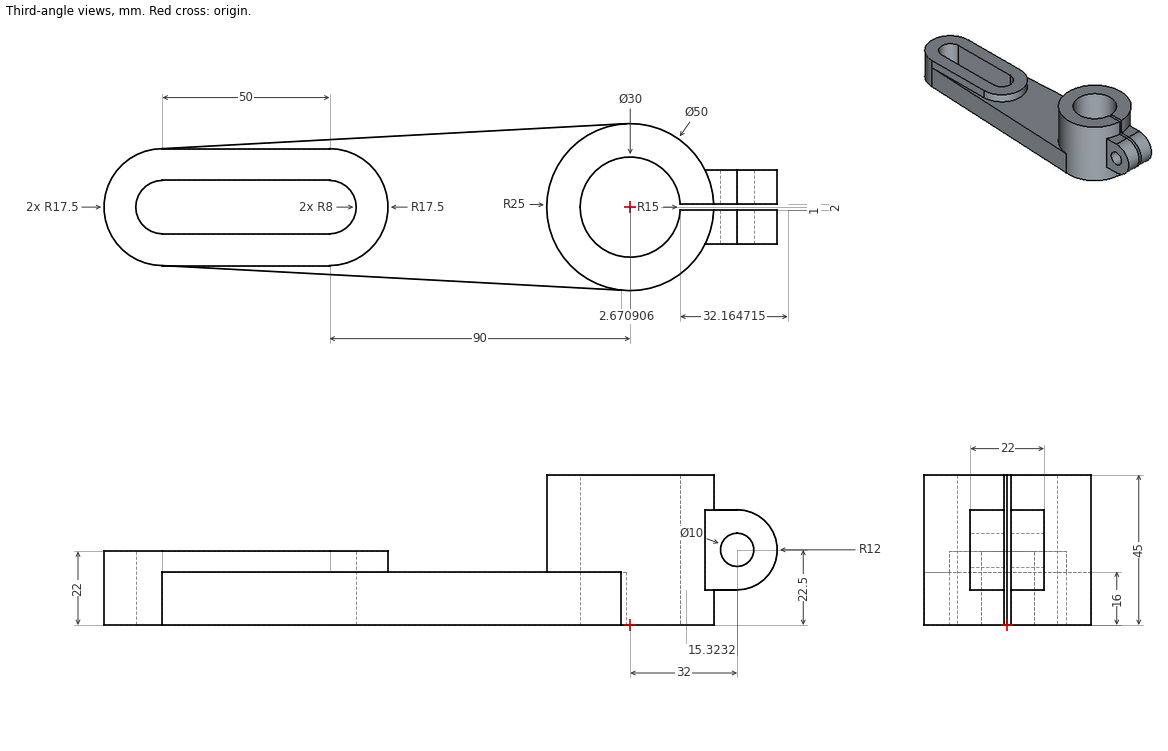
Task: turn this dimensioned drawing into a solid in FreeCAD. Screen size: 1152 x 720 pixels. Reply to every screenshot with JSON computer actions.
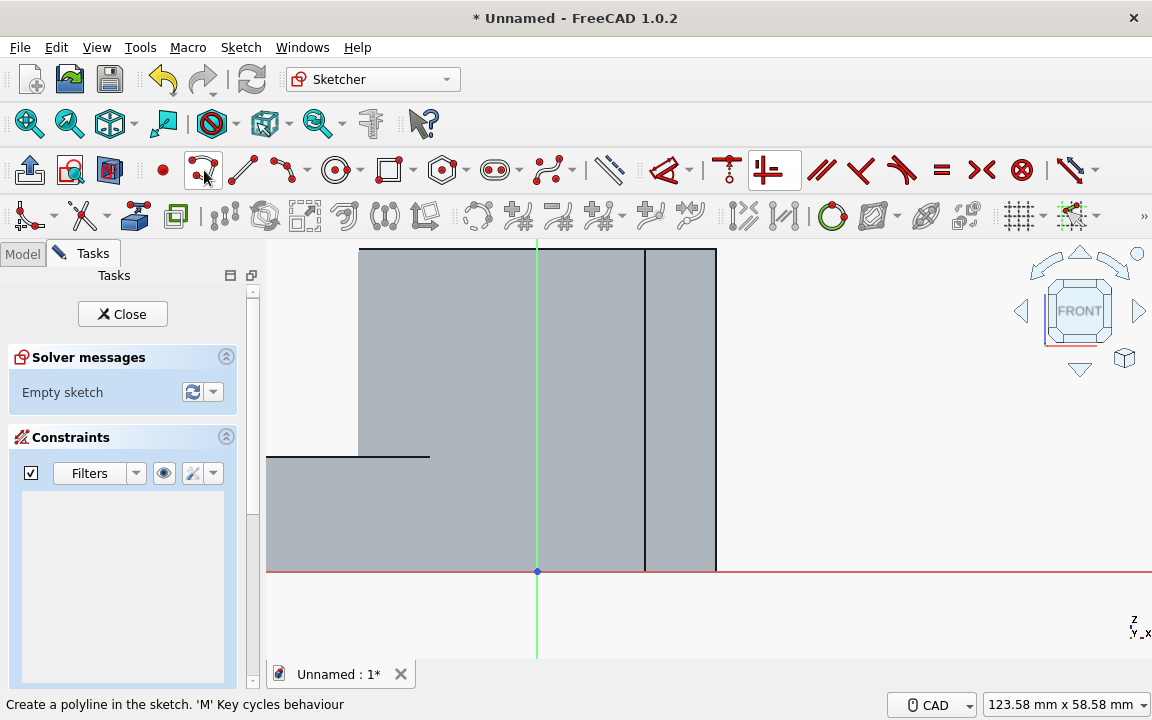
{"action": "left_click", "coordinate": [767, 497]}
{"action": "left_click", "coordinate": [657, 497]}
{"action": "left_click", "coordinate": [657, 325]}
{"action": "left_click", "coordinate": [767, 325]}
{"action": "right_click", "coordinate": [767, 325]}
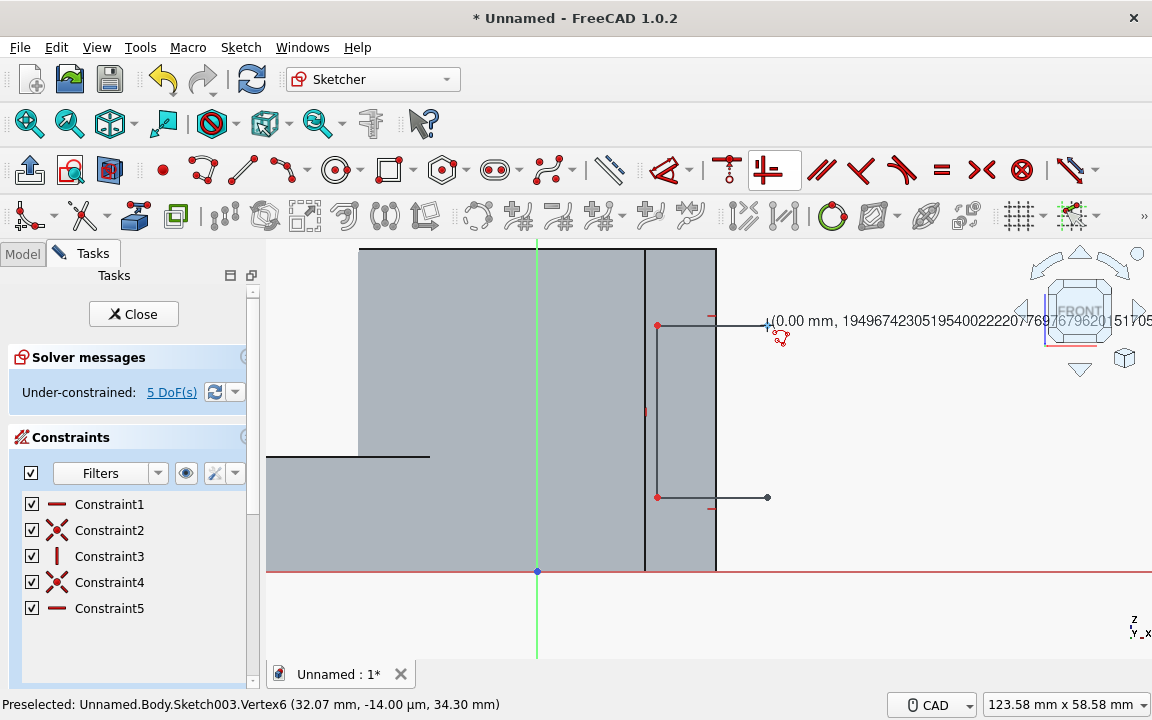
{"action": "left_click", "coordinate": [284, 170]}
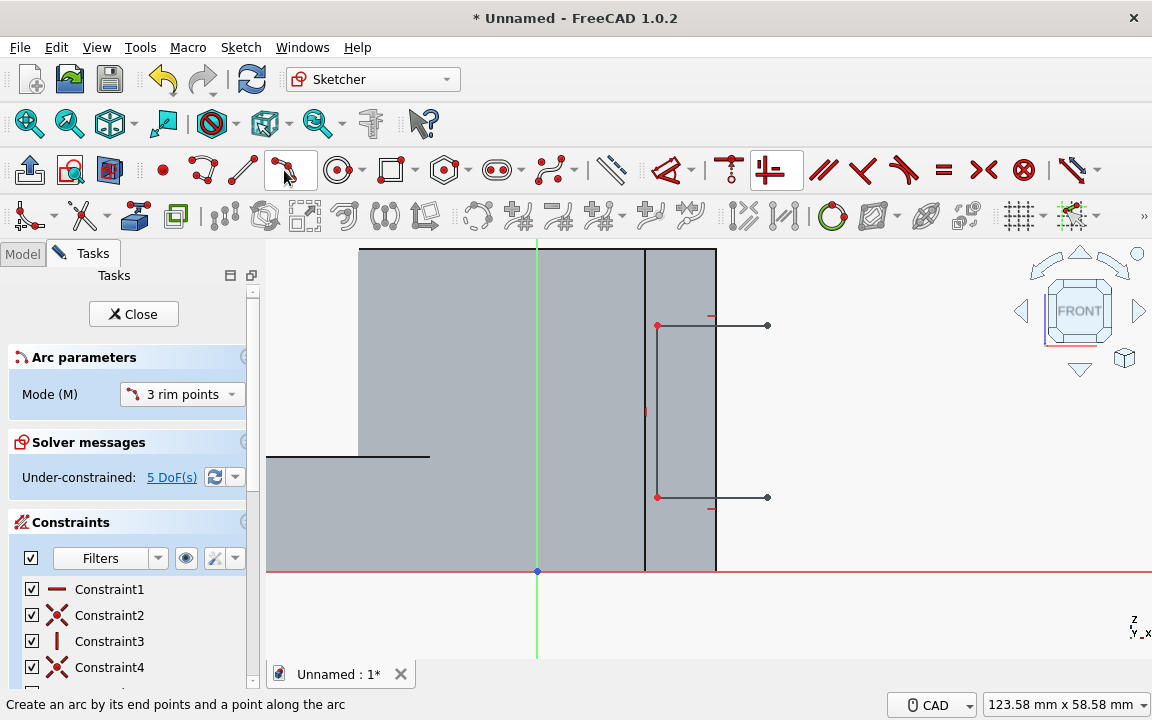
{"action": "left_click", "coordinate": [767, 326]}
{"action": "left_click", "coordinate": [767, 498]}
{"action": "left_click", "coordinate": [853, 411]}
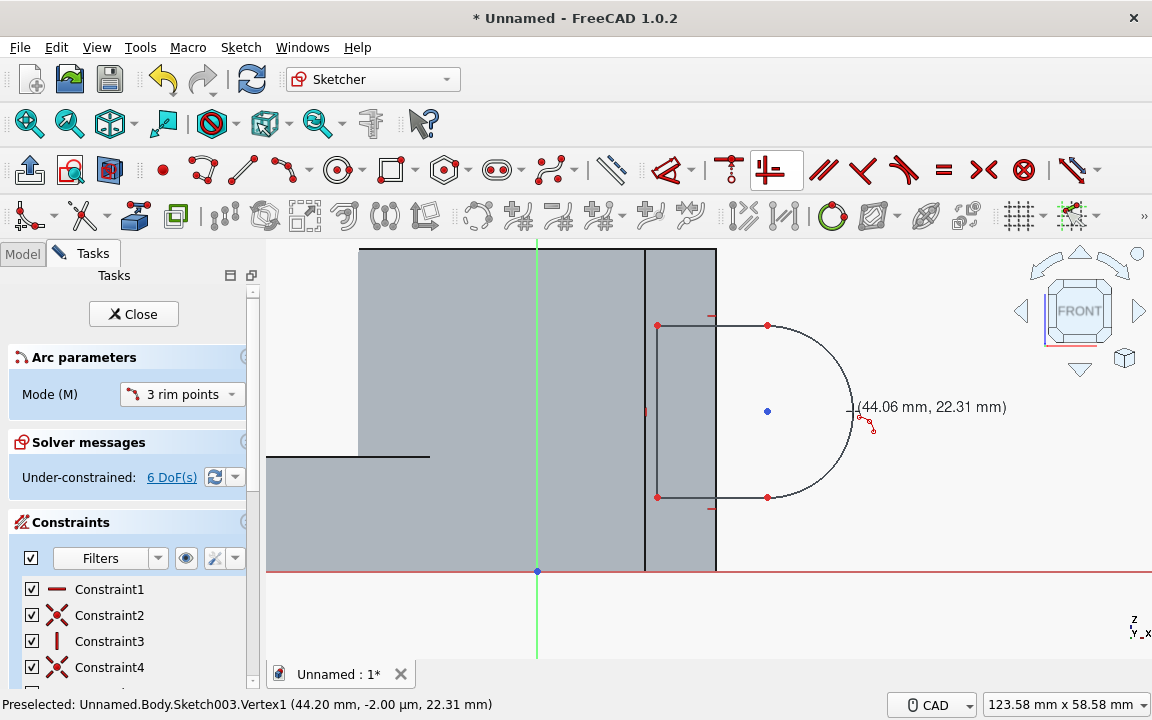
{"action": "left_click", "coordinate": [338, 170]}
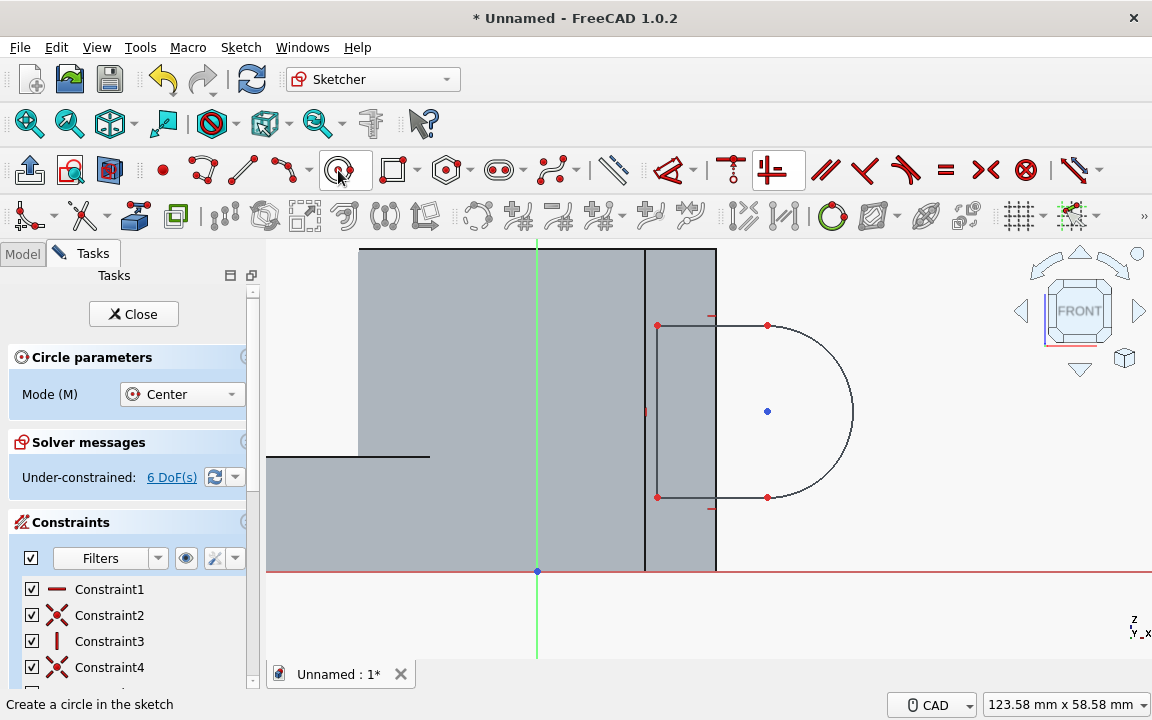
{"action": "left_click", "coordinate": [767, 411]}
{"action": "left_click", "coordinate": [792, 385]}
{"action": "key", "text": "Escape"}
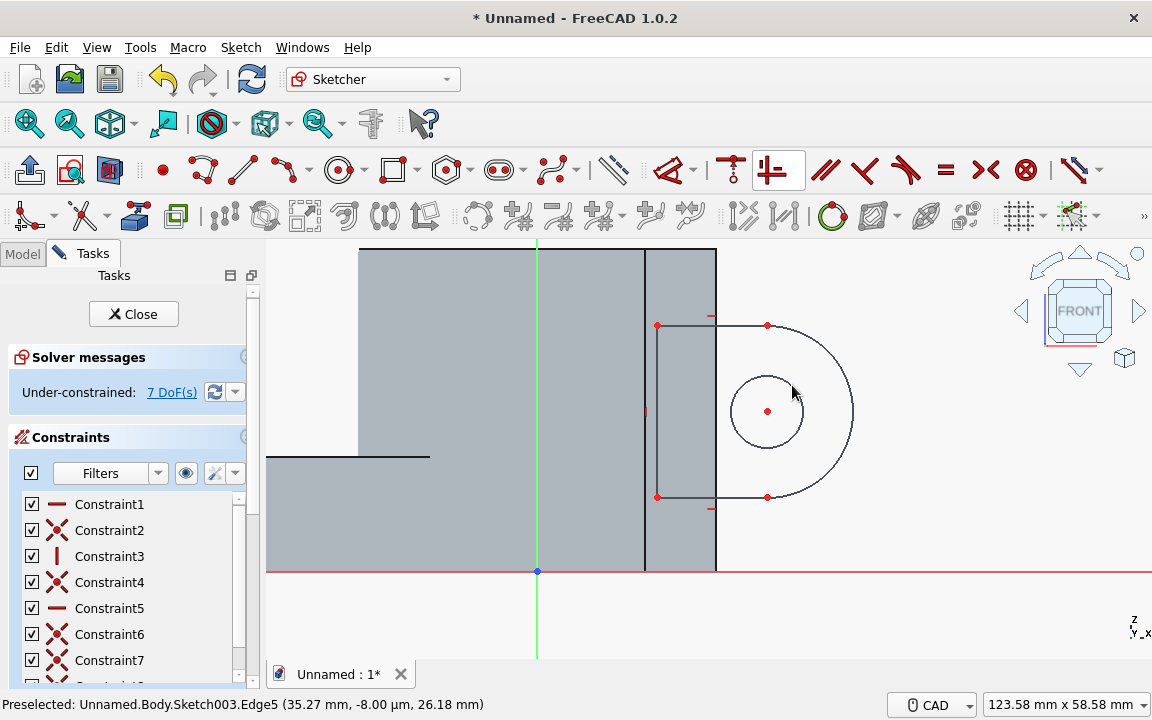
{"action": "left_click", "coordinate": [734, 498]}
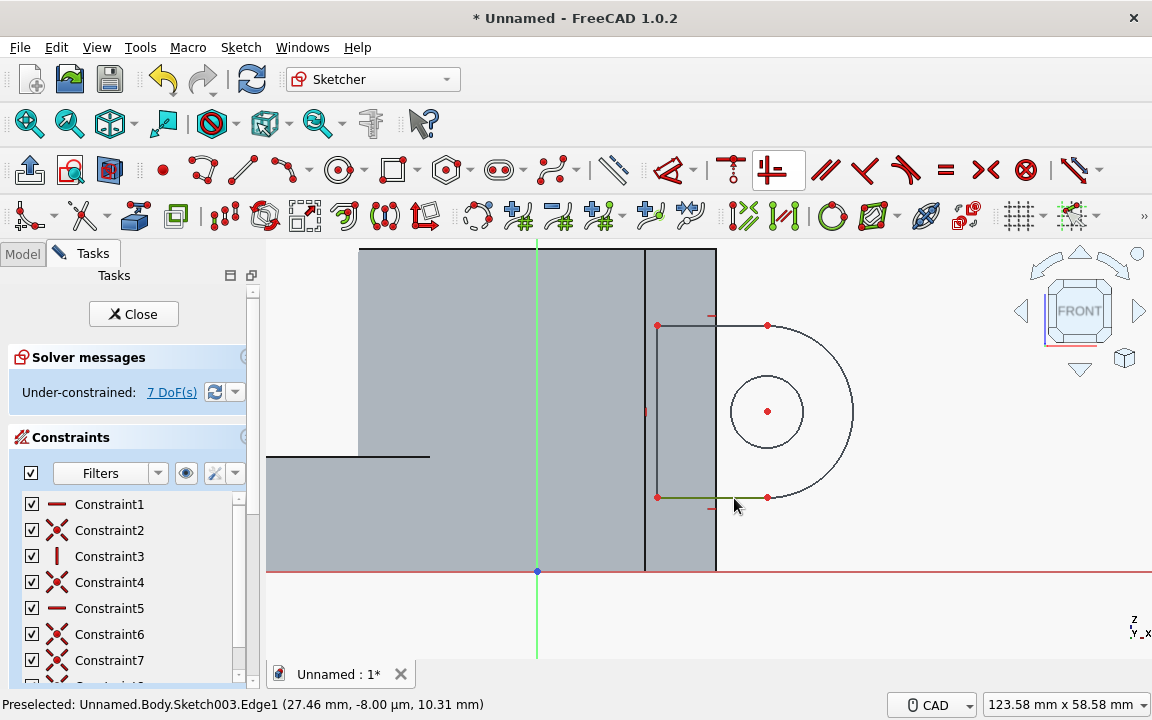
{"action": "left_click", "coordinate": [837, 463]}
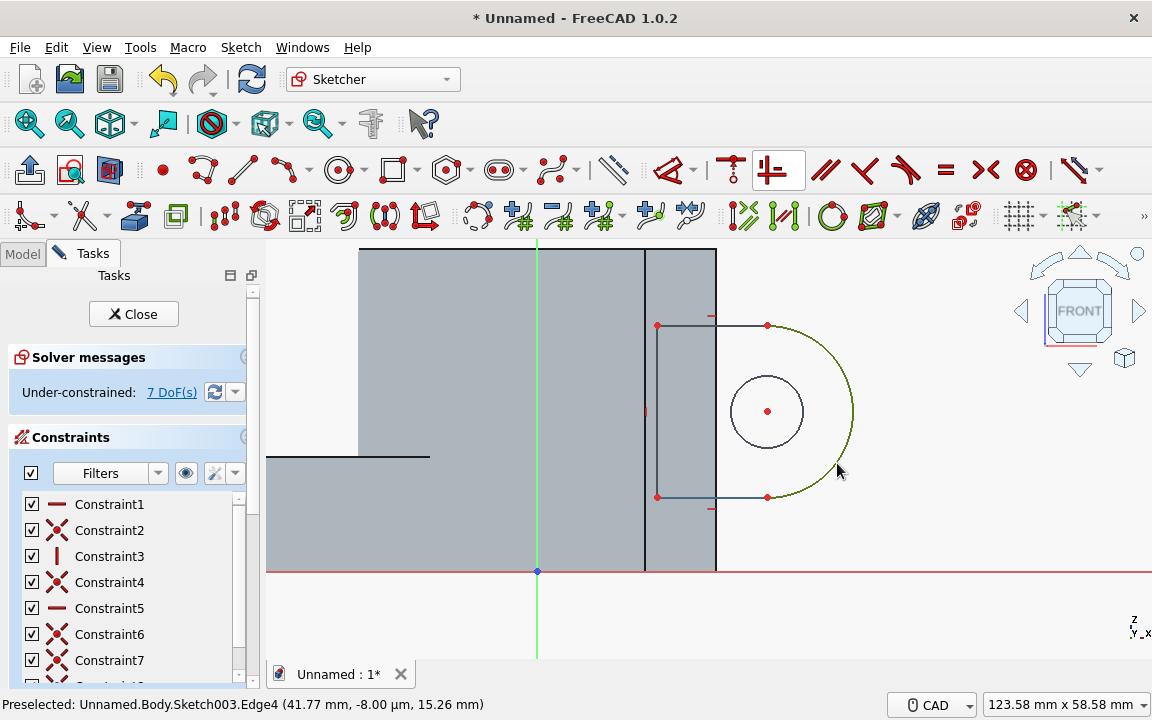
{"action": "left_click", "coordinate": [906, 170]}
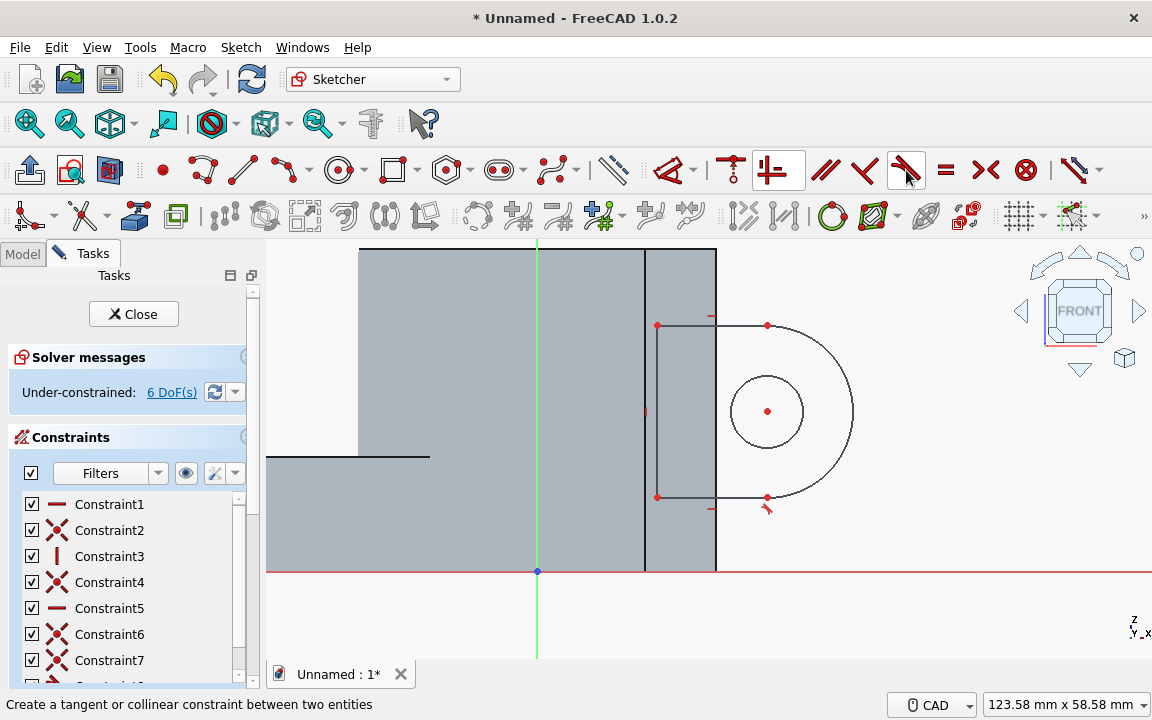
{"action": "left_click", "coordinate": [690, 326]}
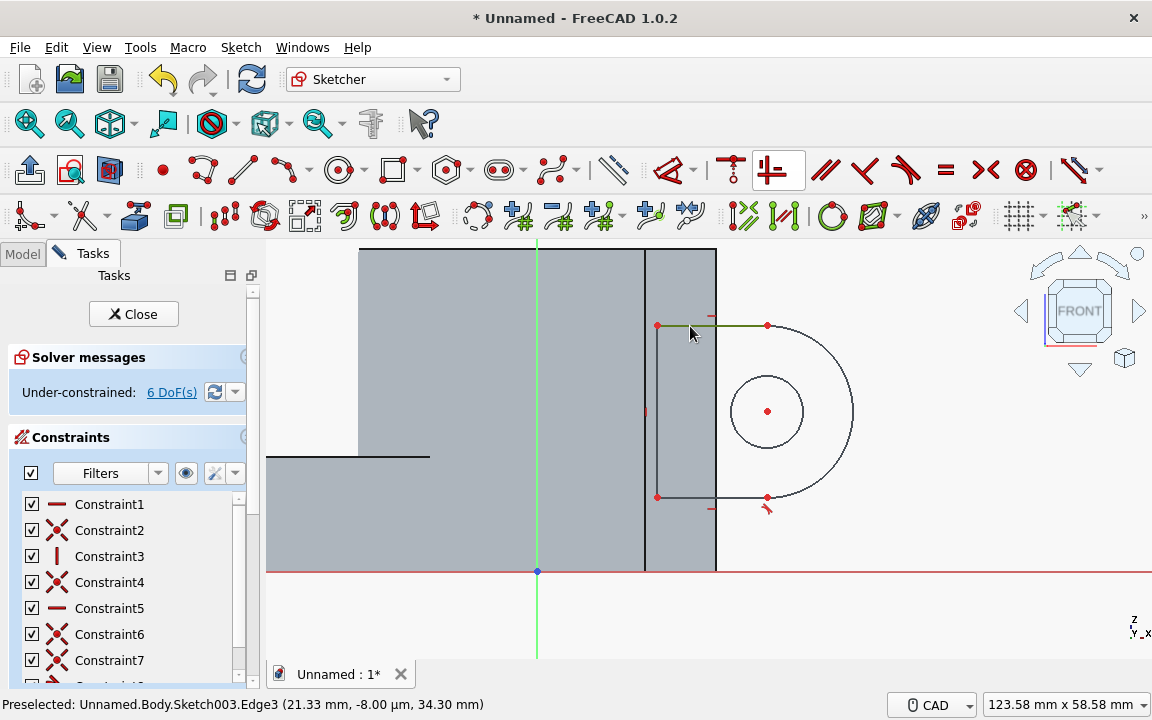
{"action": "left_click", "coordinate": [837, 463]}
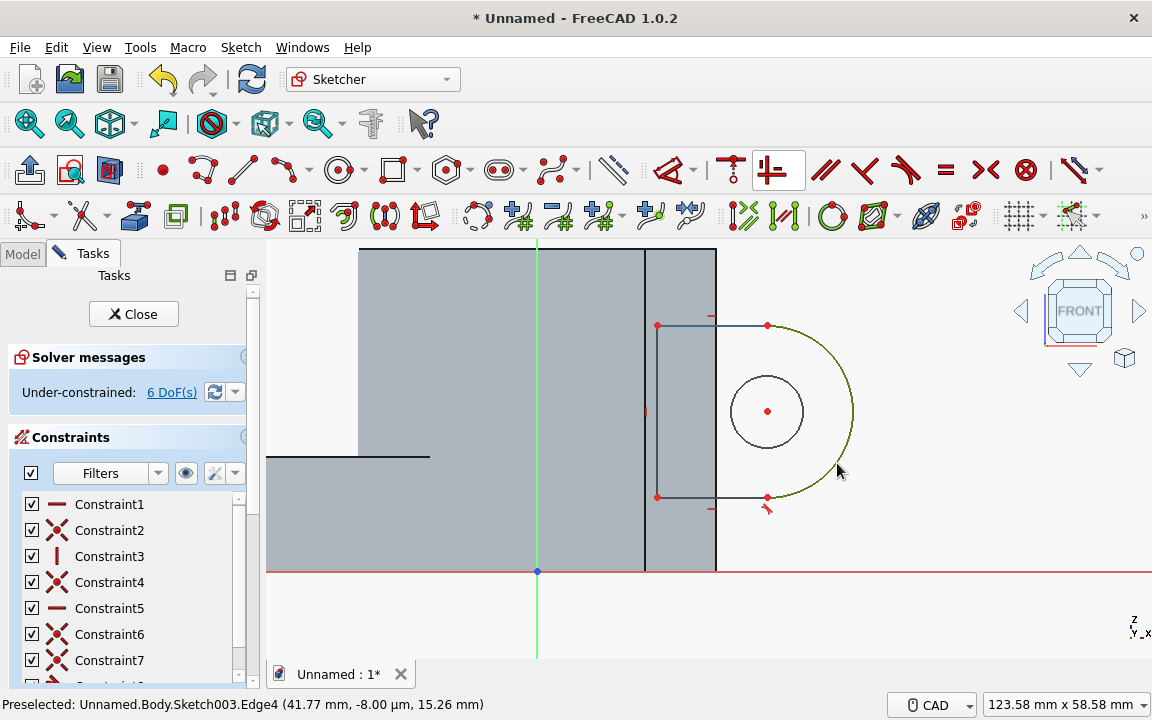
{"action": "left_click", "coordinate": [906, 170]}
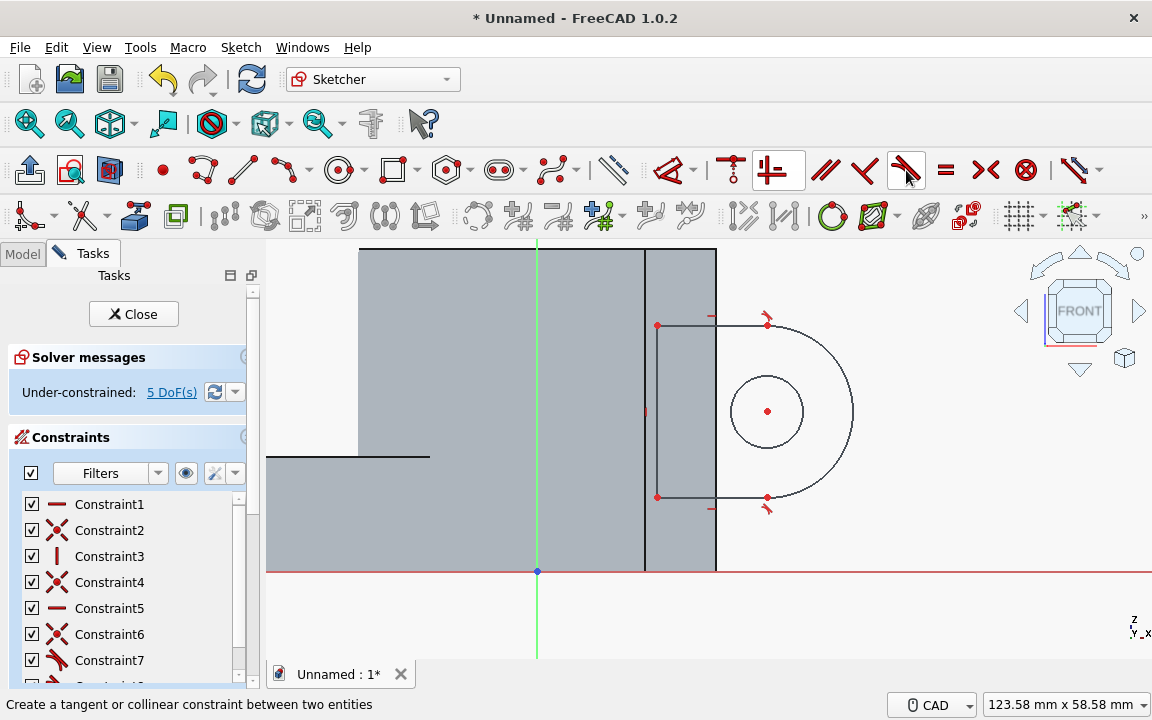
{"action": "key", "text": "d"}